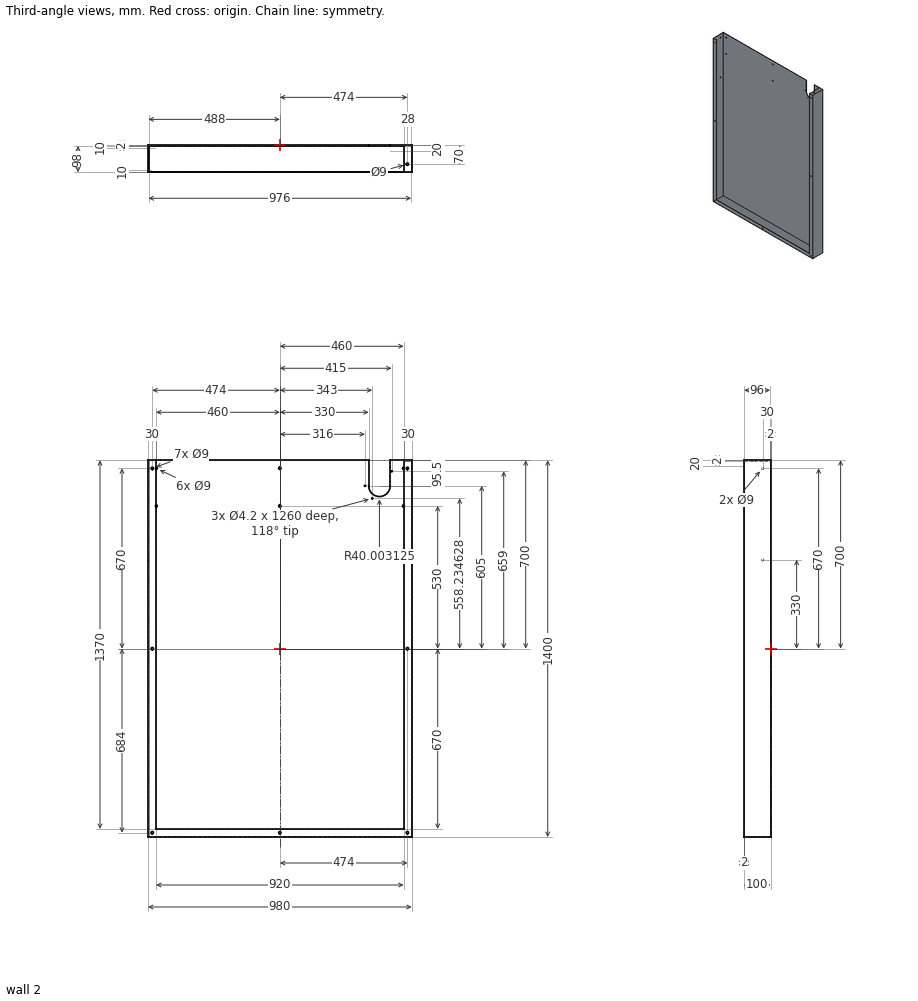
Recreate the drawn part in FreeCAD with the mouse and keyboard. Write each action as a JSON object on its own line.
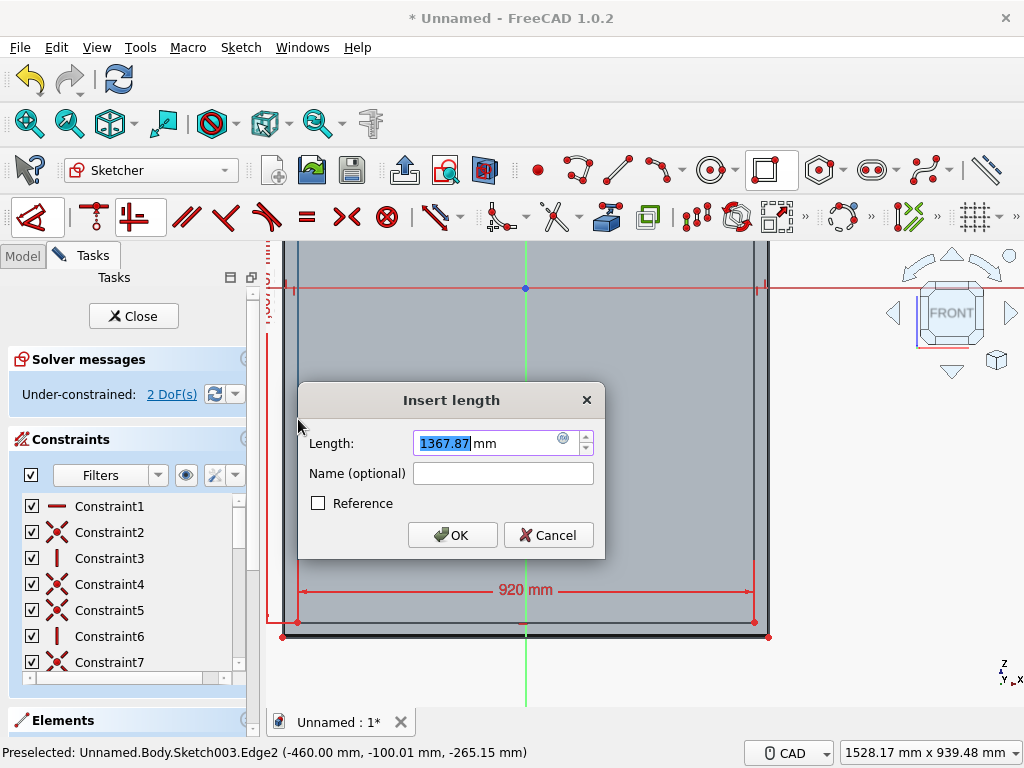
{"action": "type", "text": "1370"}
{"action": "key", "text": "Return"}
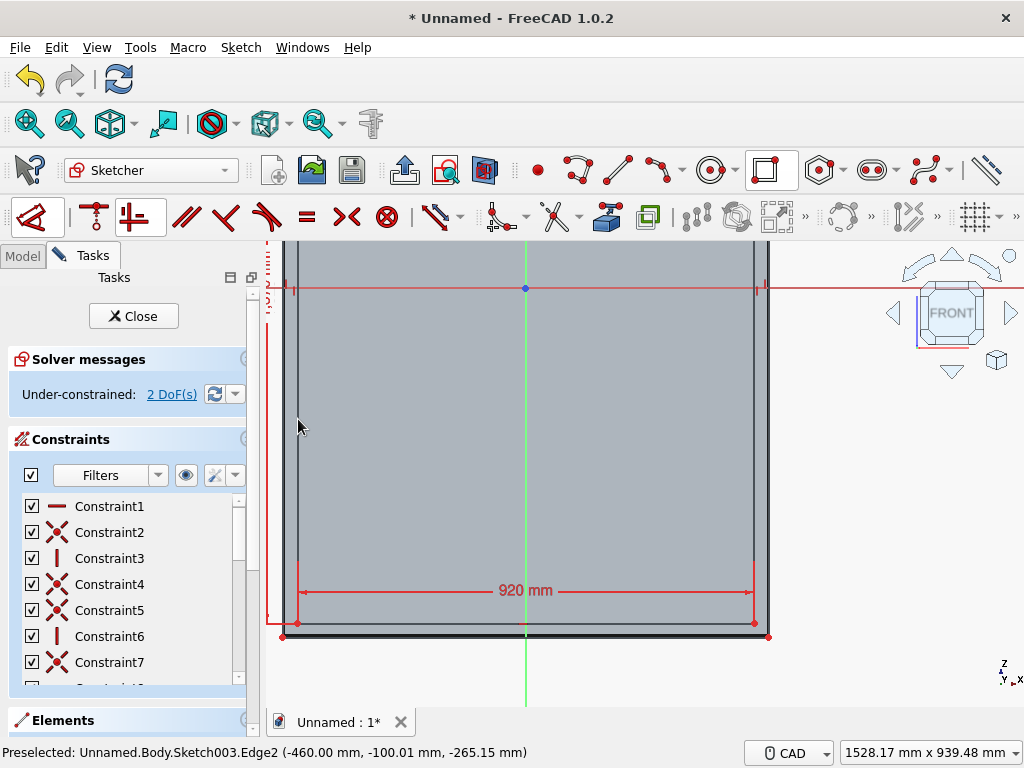
{"action": "scroll", "coordinate": [618, 625], "scroll_direction": "down", "scroll_amount": 4}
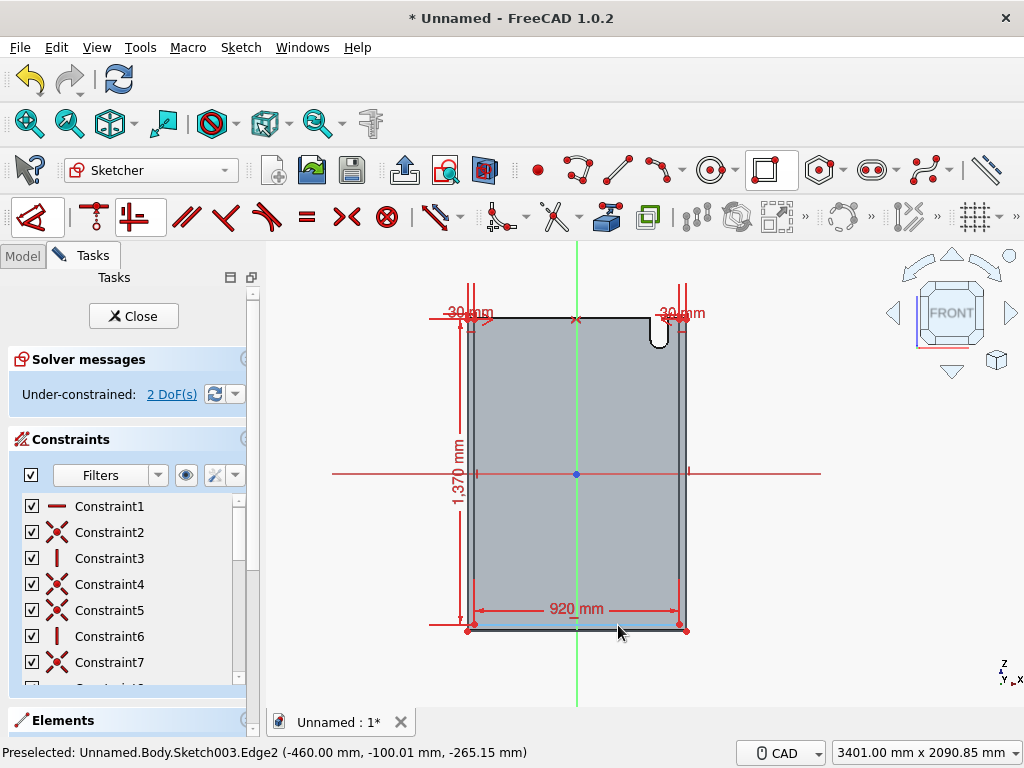
{"action": "scroll", "coordinate": [468, 413], "scroll_direction": "up", "scroll_amount": 4}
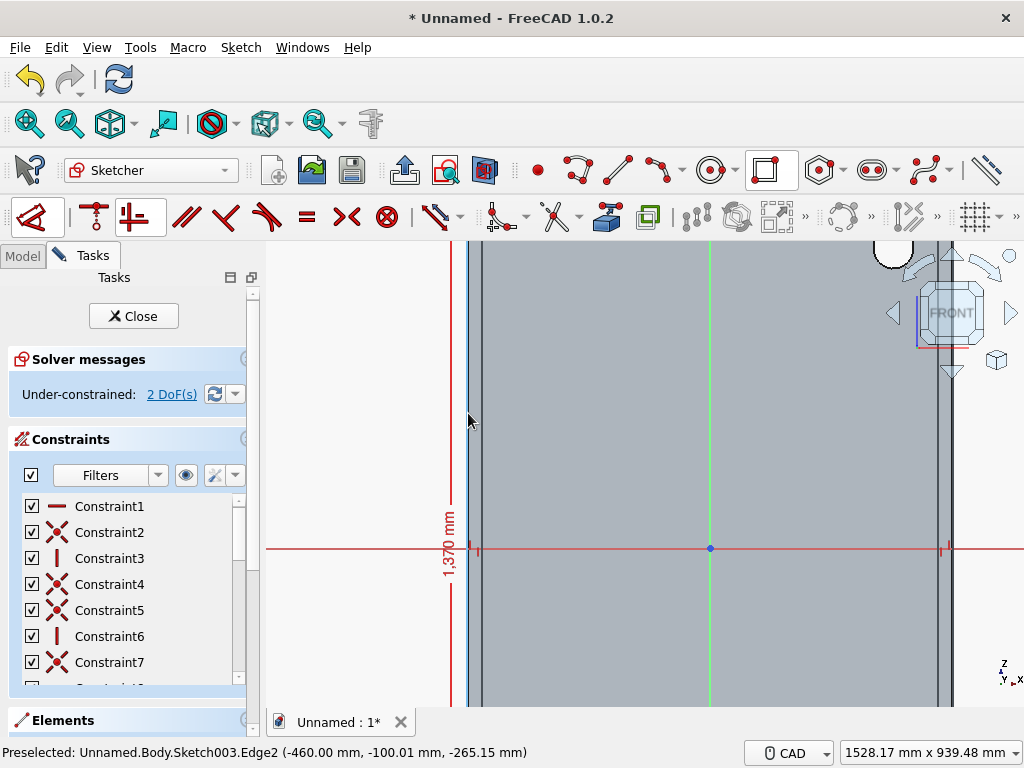
{"action": "left_click", "coordinate": [467, 412]}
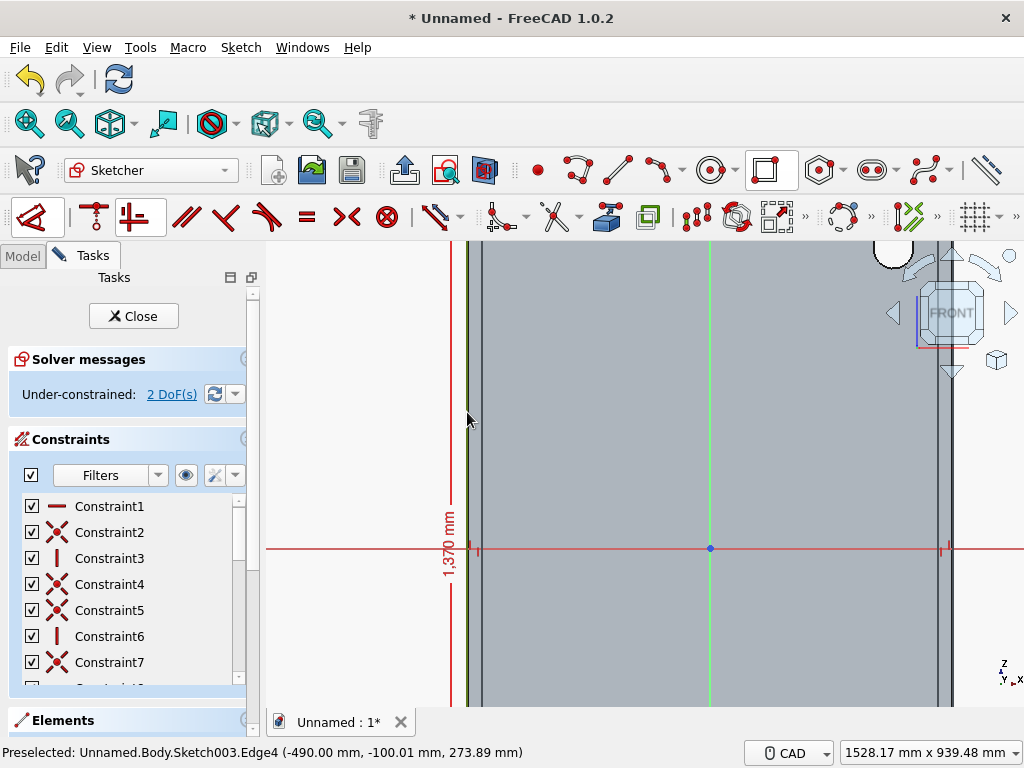
{"action": "left_click", "coordinate": [58, 218]}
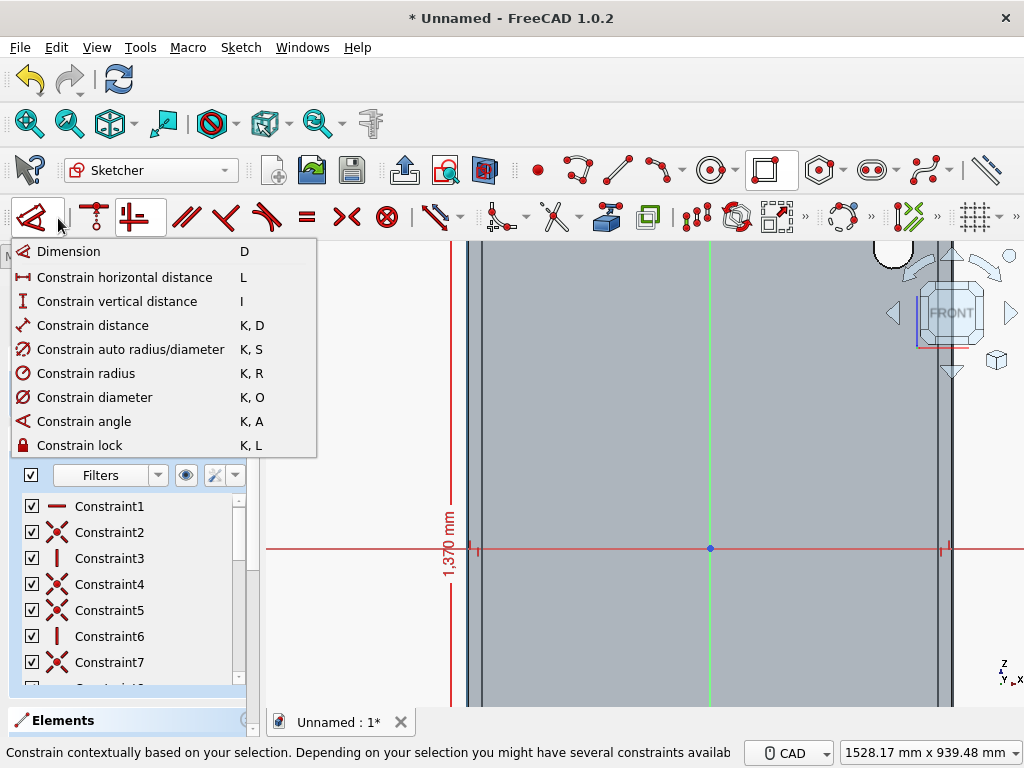
{"action": "left_click", "coordinate": [164, 301]}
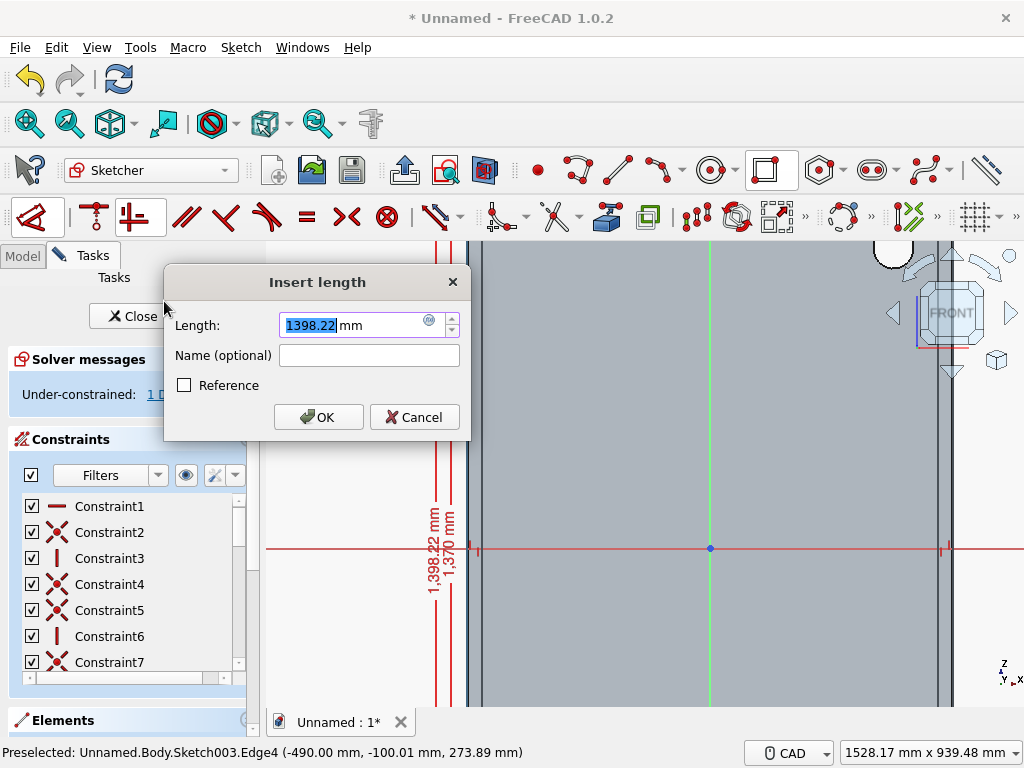
{"action": "type", "text": "1400"}
{"action": "key", "text": "Return"}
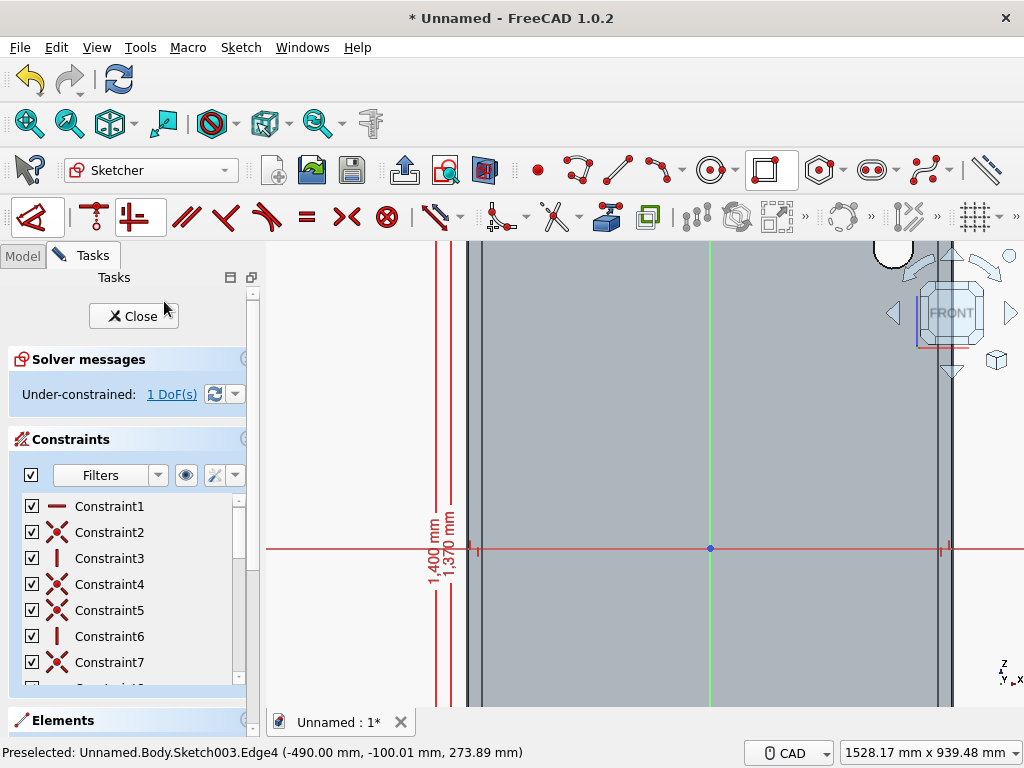
{"action": "scroll", "coordinate": [468, 413], "scroll_direction": "down", "scroll_amount": 4}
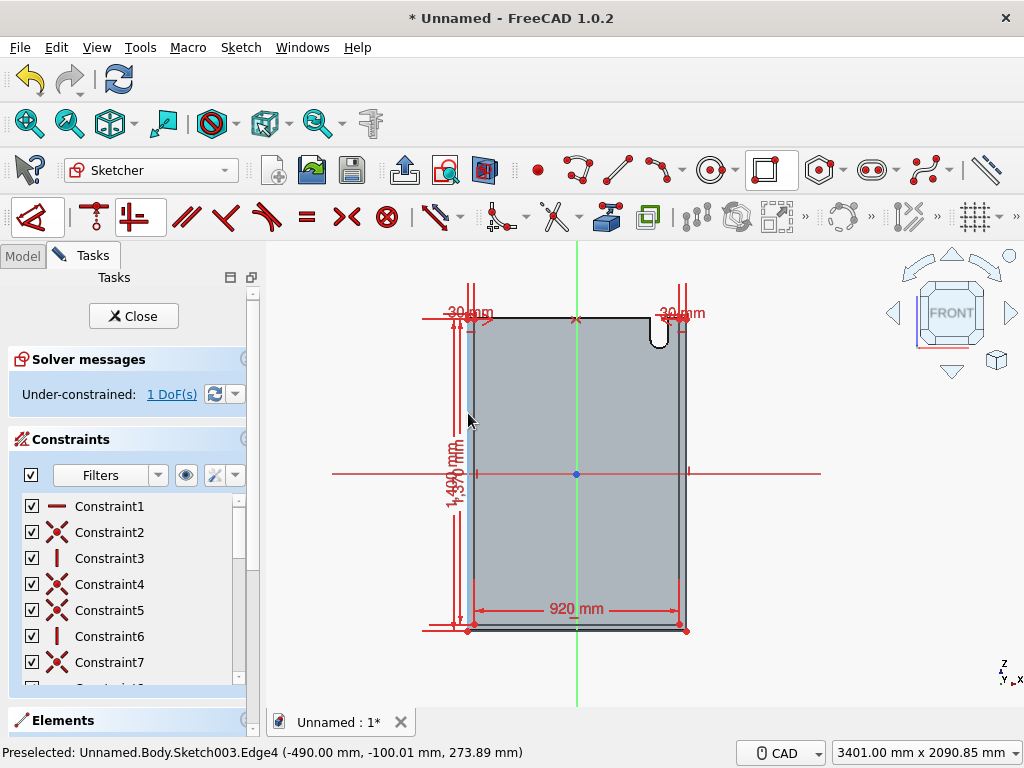
{"action": "scroll", "coordinate": [679, 625], "scroll_direction": "up", "scroll_amount": 2}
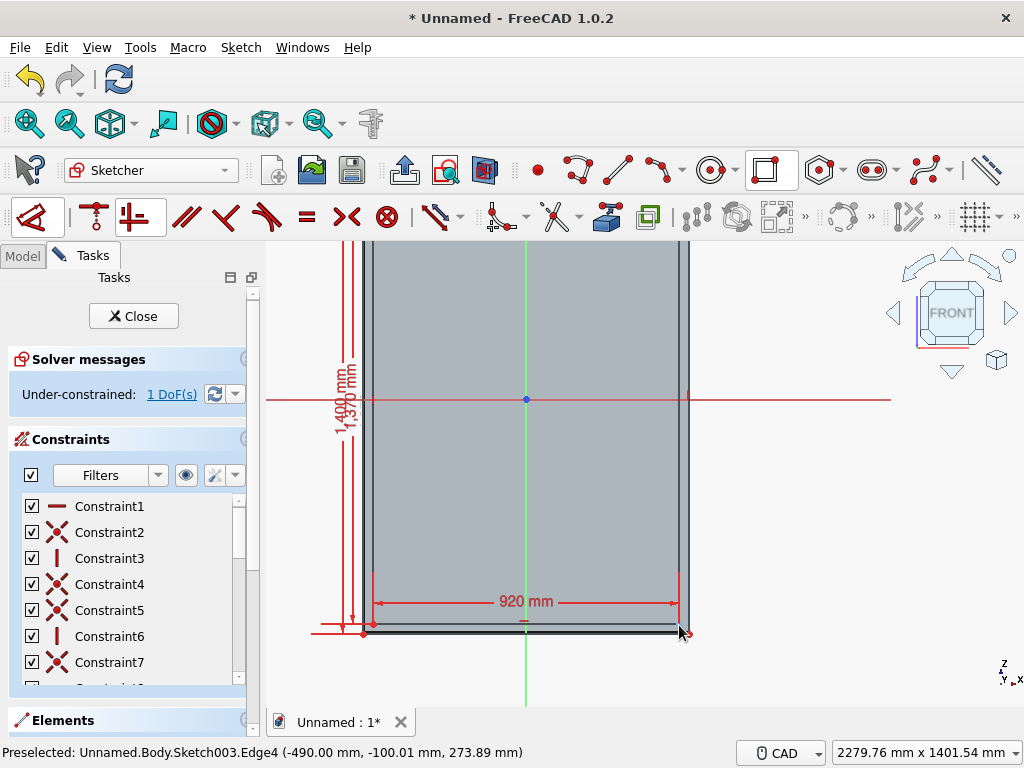
{"action": "left_click", "coordinate": [679, 624]}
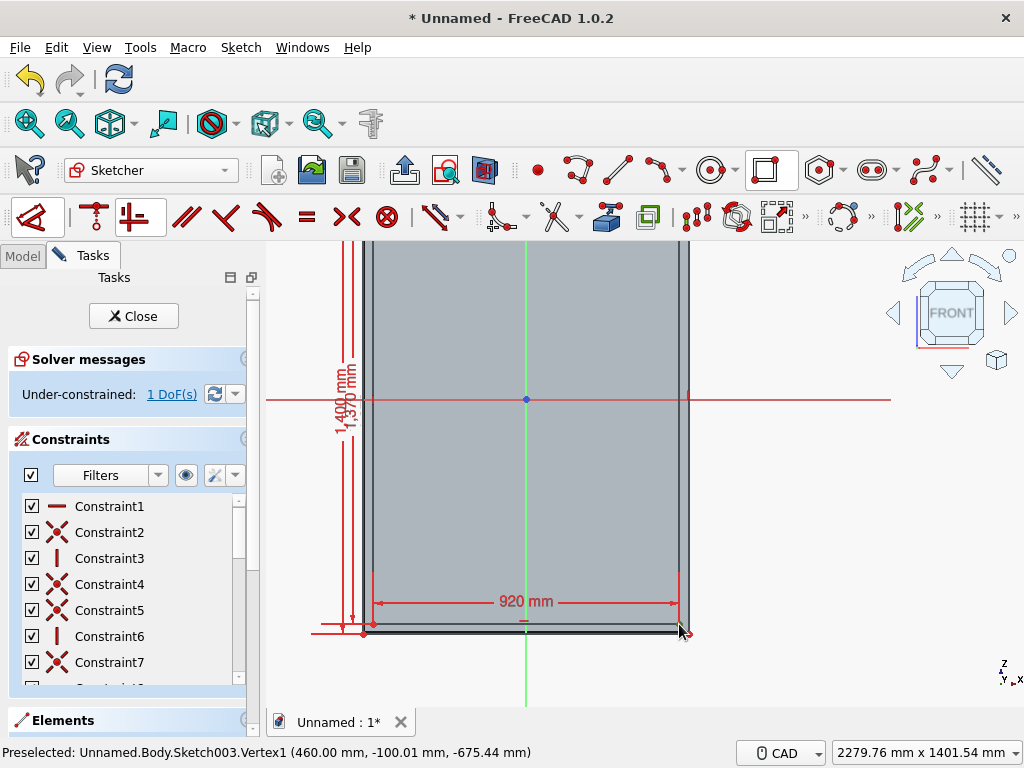
{"action": "left_click", "coordinate": [58, 218]}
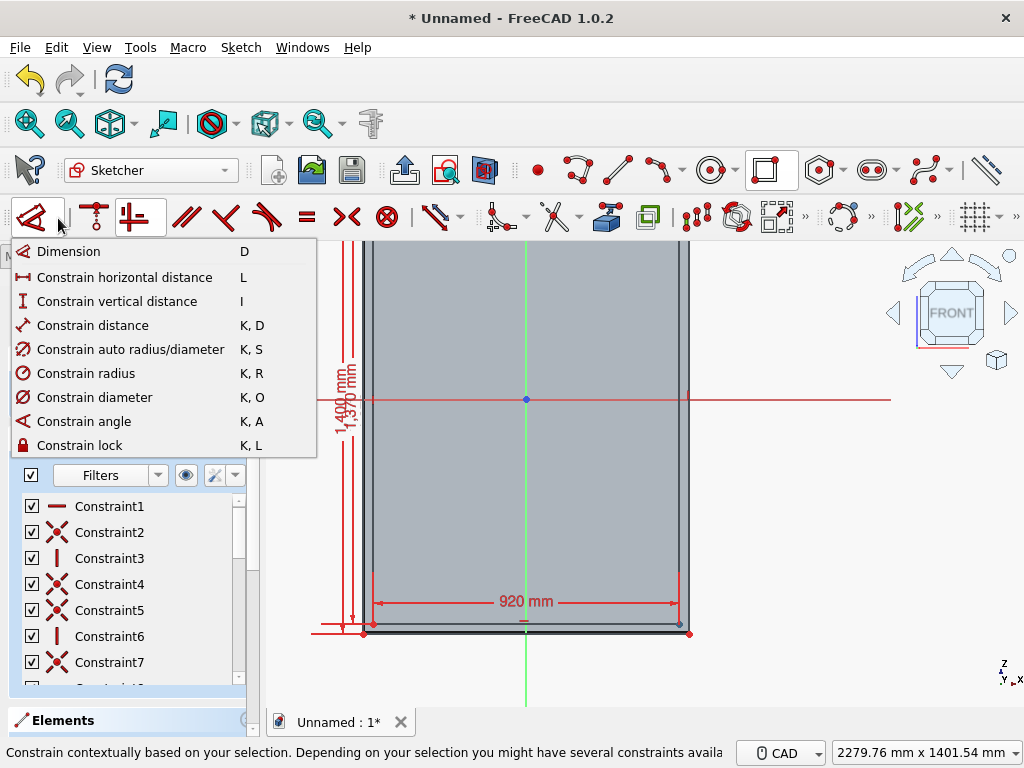
{"action": "left_click", "coordinate": [164, 301]}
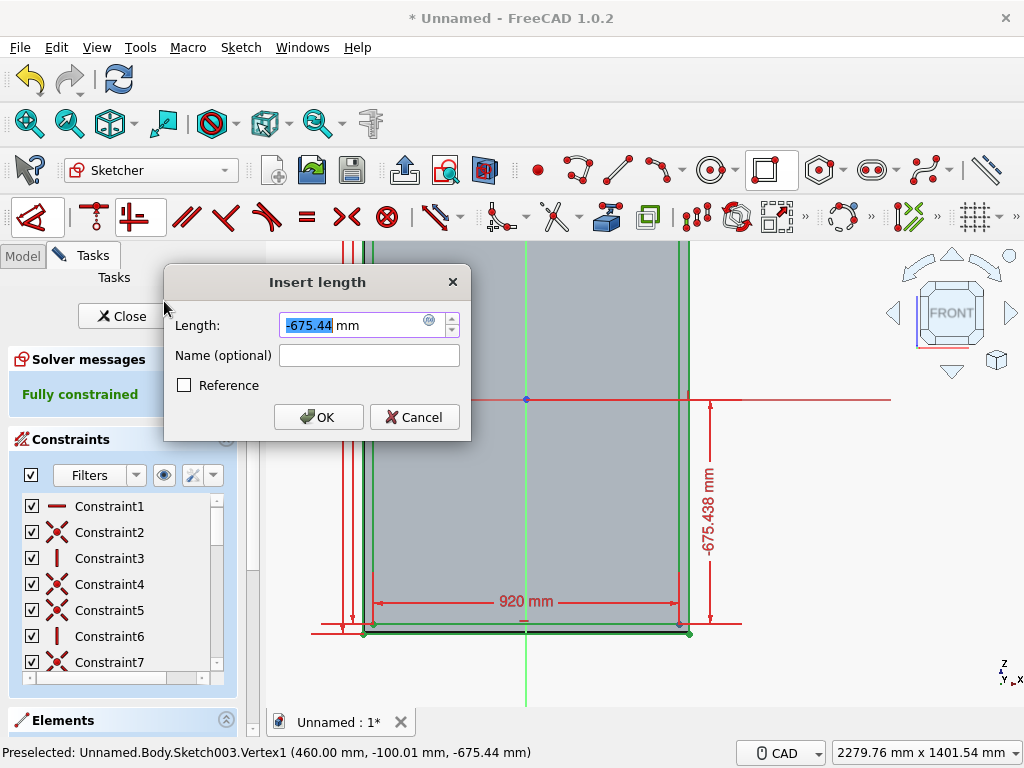
{"action": "type", "text": "-670"}
{"action": "key", "text": "Return"}